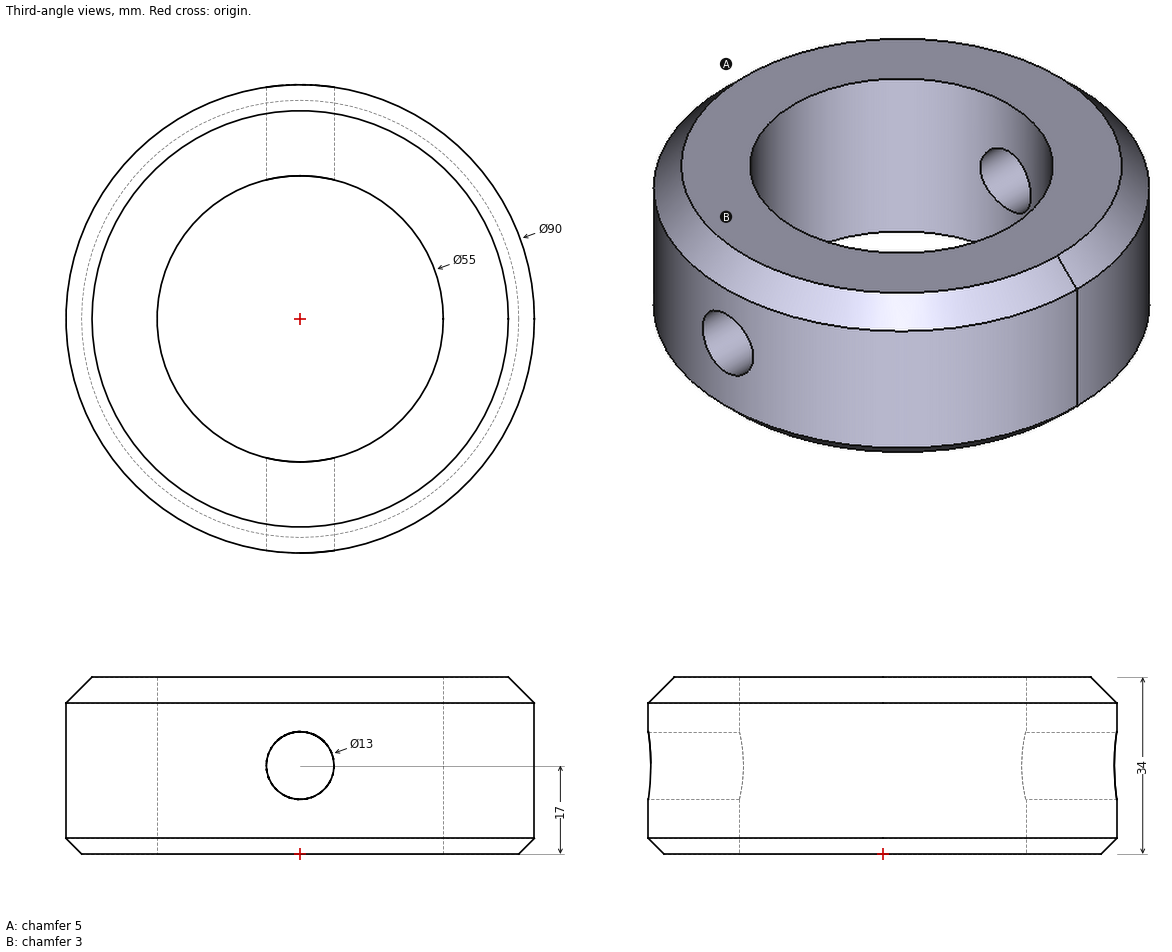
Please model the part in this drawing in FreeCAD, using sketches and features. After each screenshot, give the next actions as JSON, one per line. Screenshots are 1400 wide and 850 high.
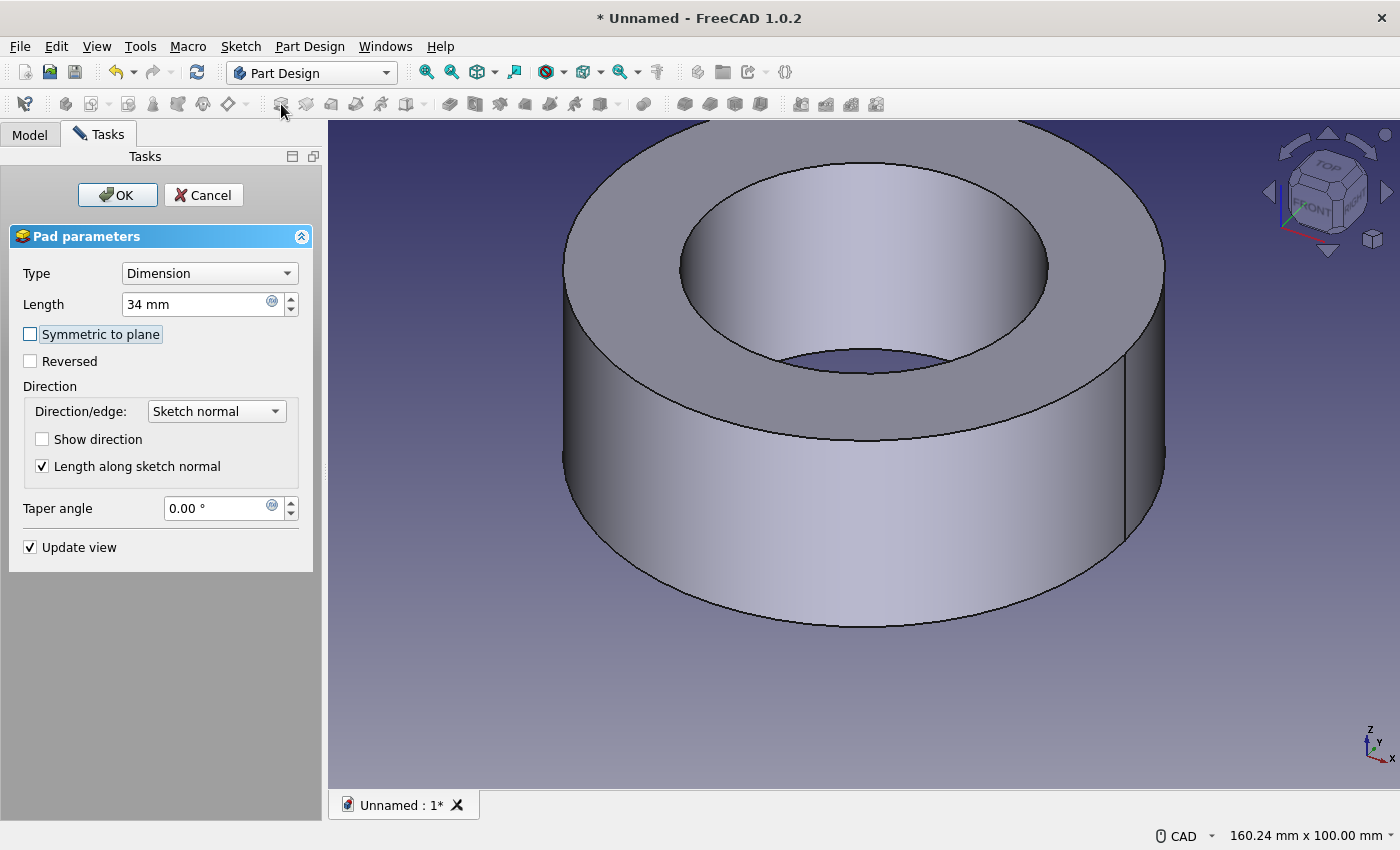
{"action": "left_click", "coordinate": [118, 195]}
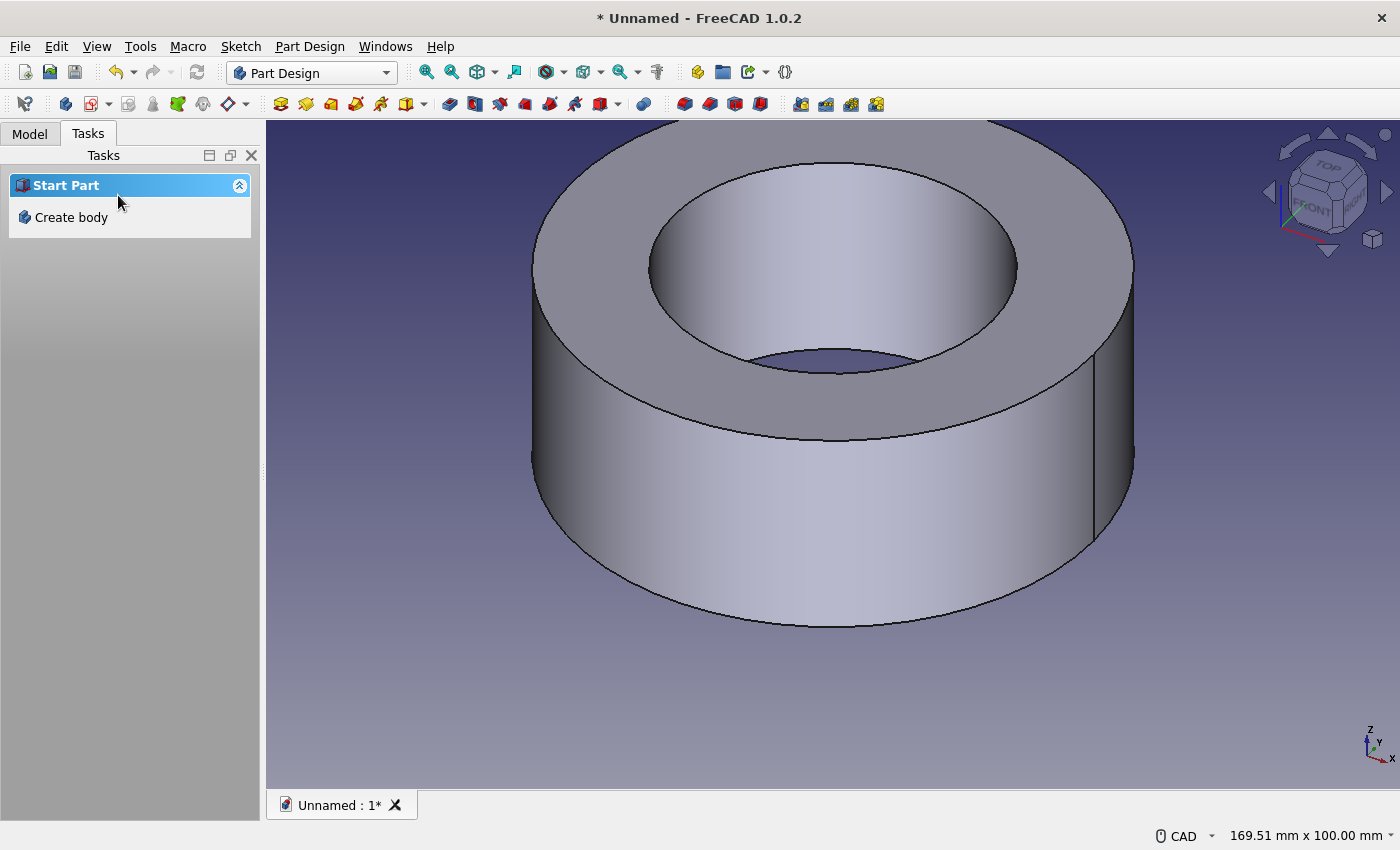
{"action": "left_click", "coordinate": [427, 72]}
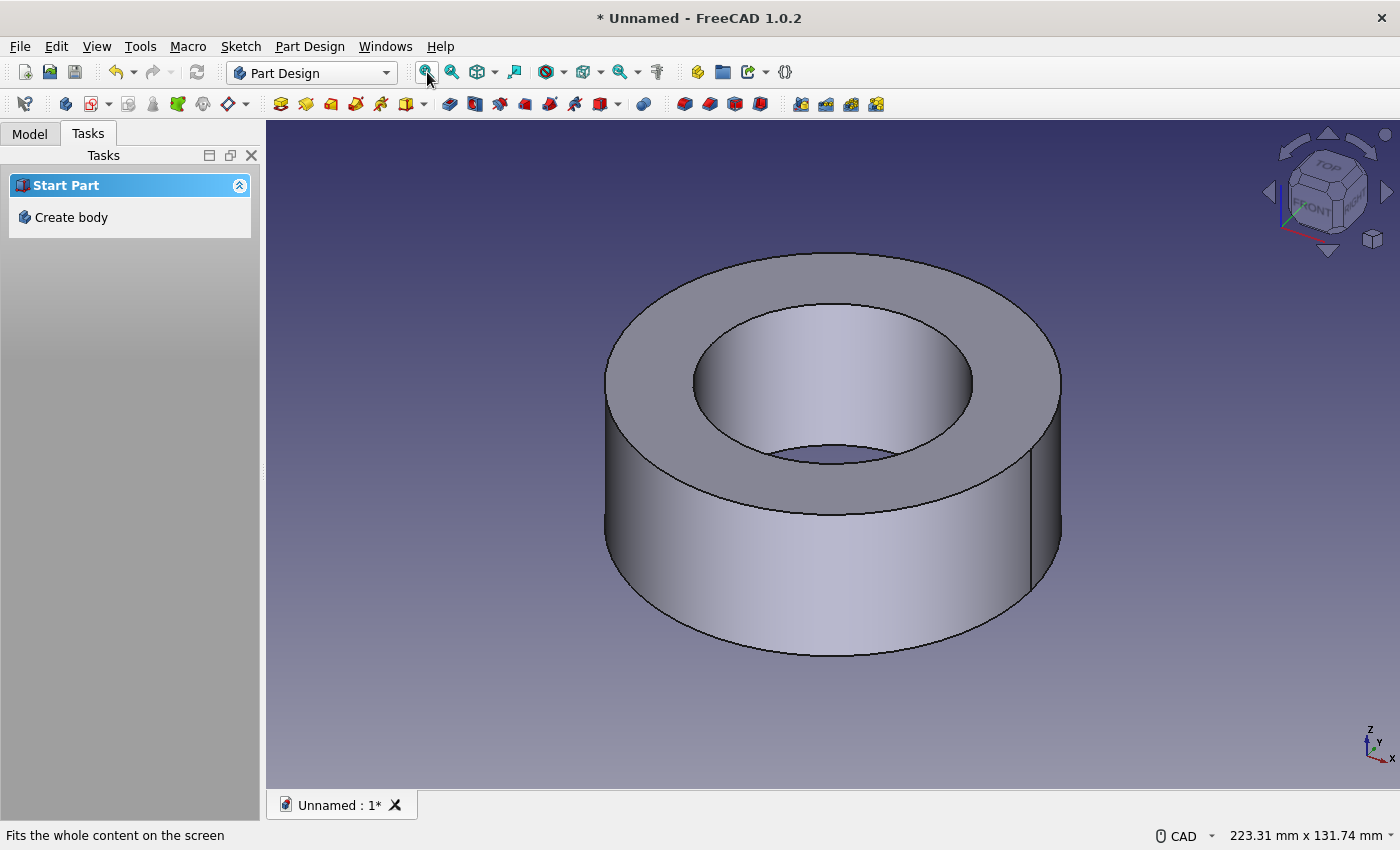
{"action": "left_click", "coordinate": [90, 104]}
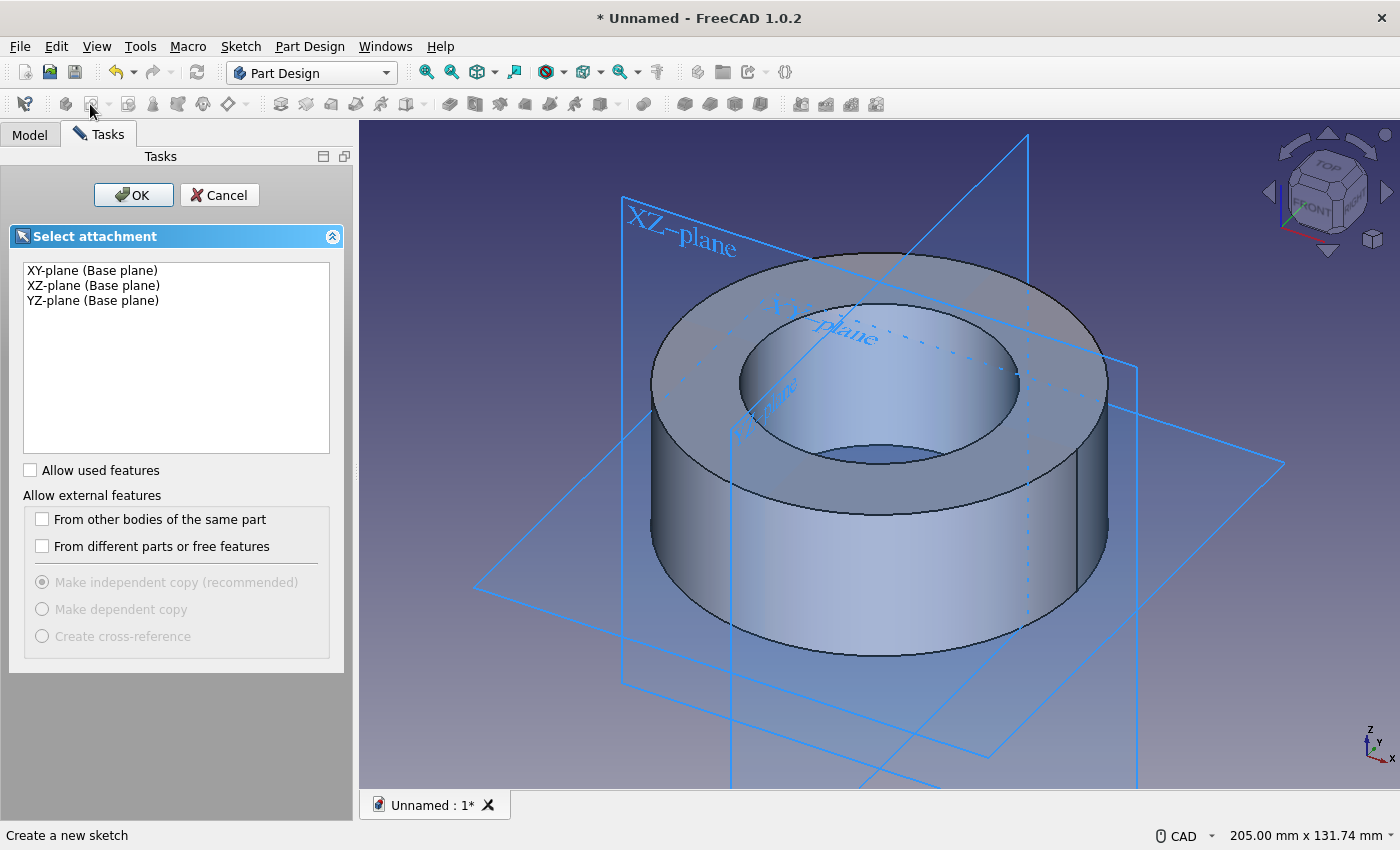
{"action": "left_click", "coordinate": [84, 286]}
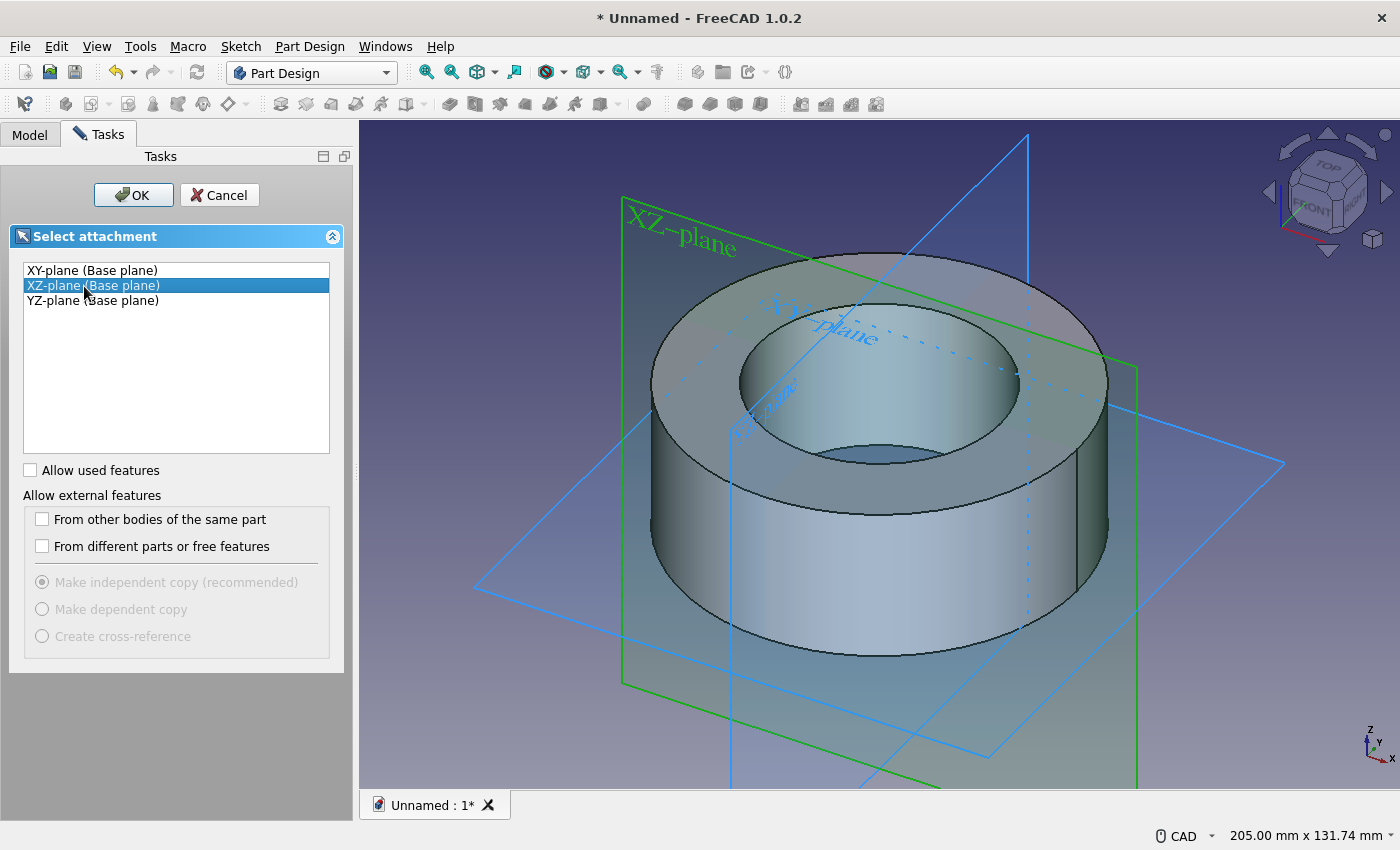
{"action": "left_click", "coordinate": [134, 195]}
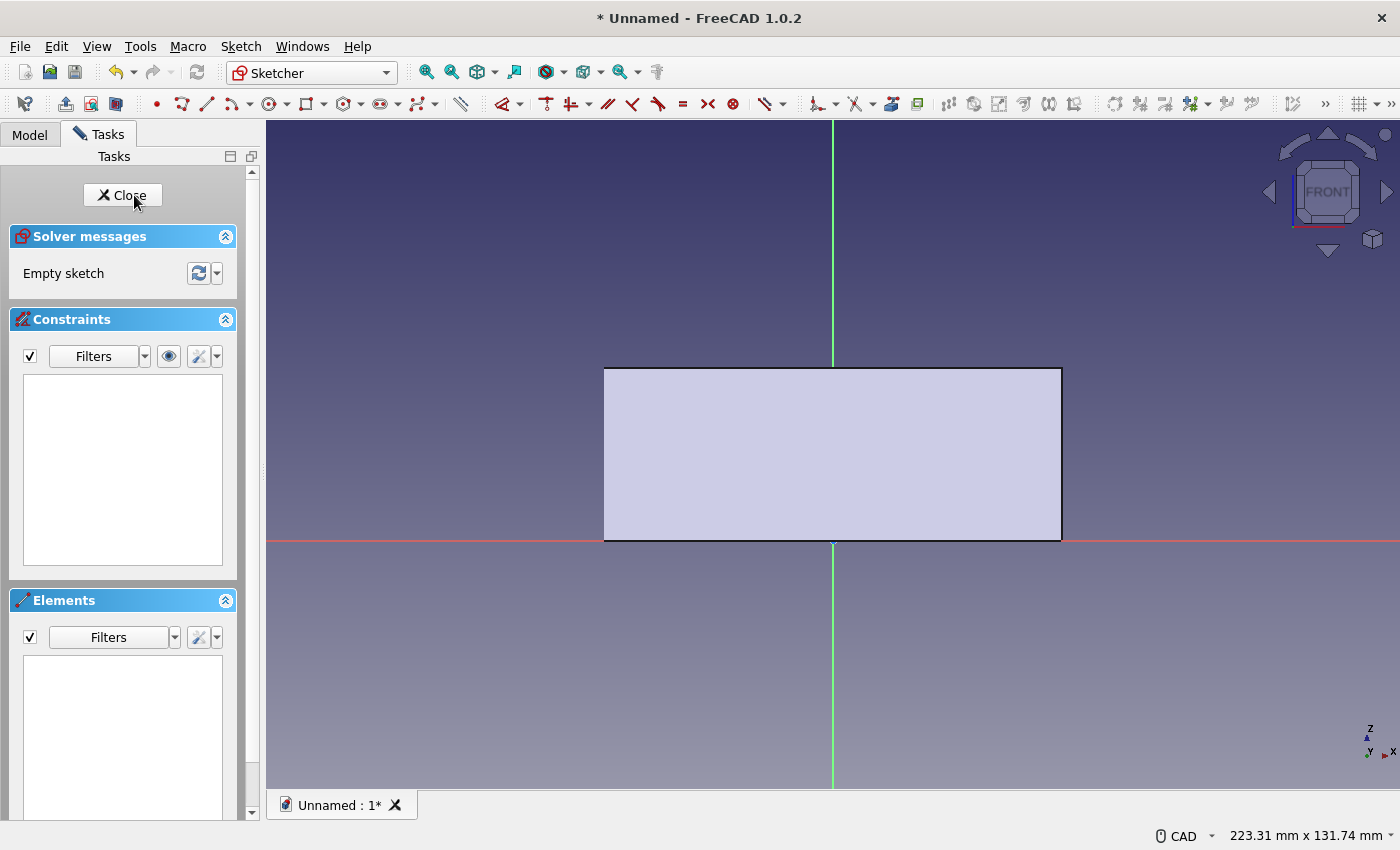
{"action": "key", "text": "q s"}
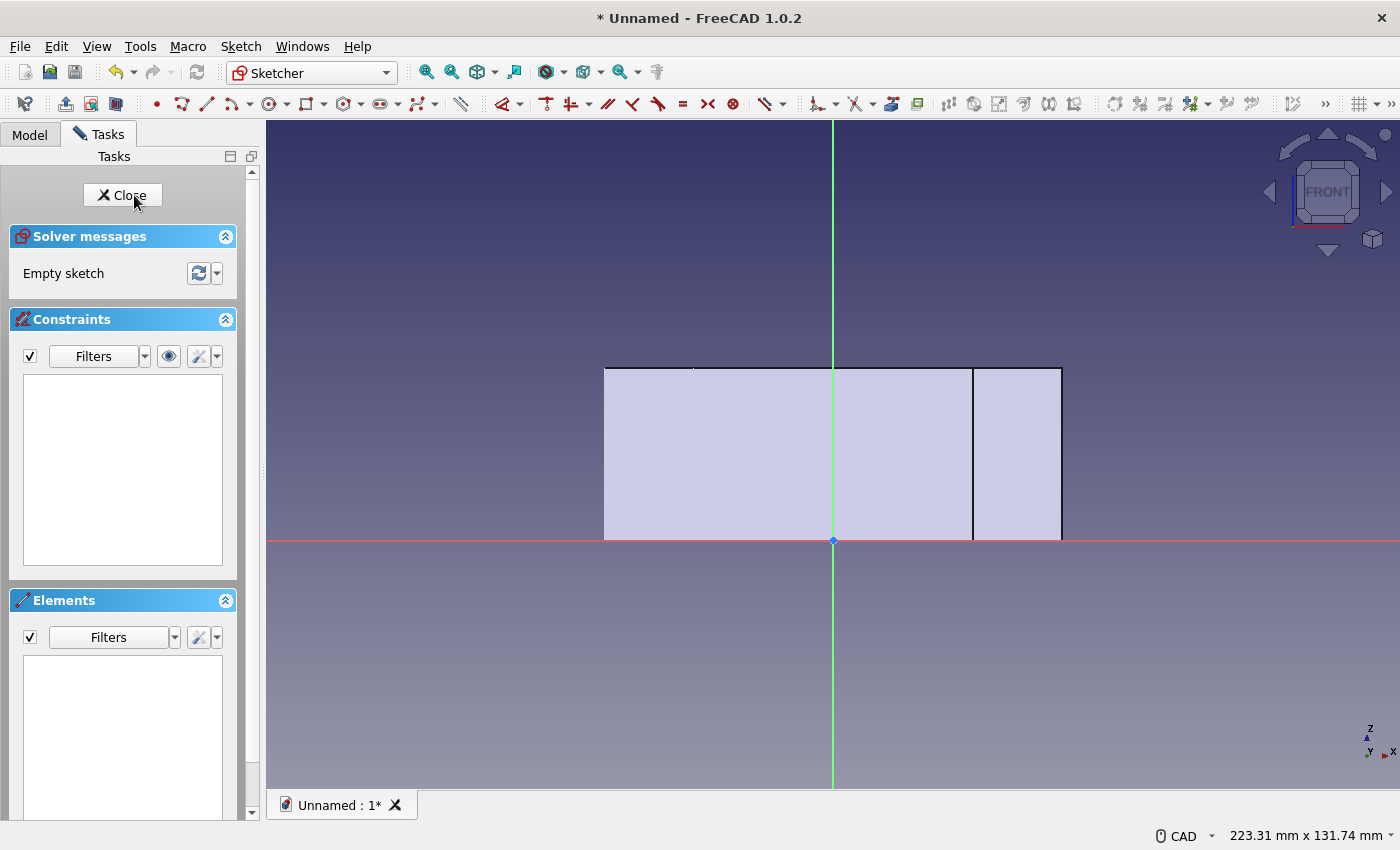
{"action": "scroll", "coordinate": [863, 493], "scroll_direction": "up", "scroll_amount": 6}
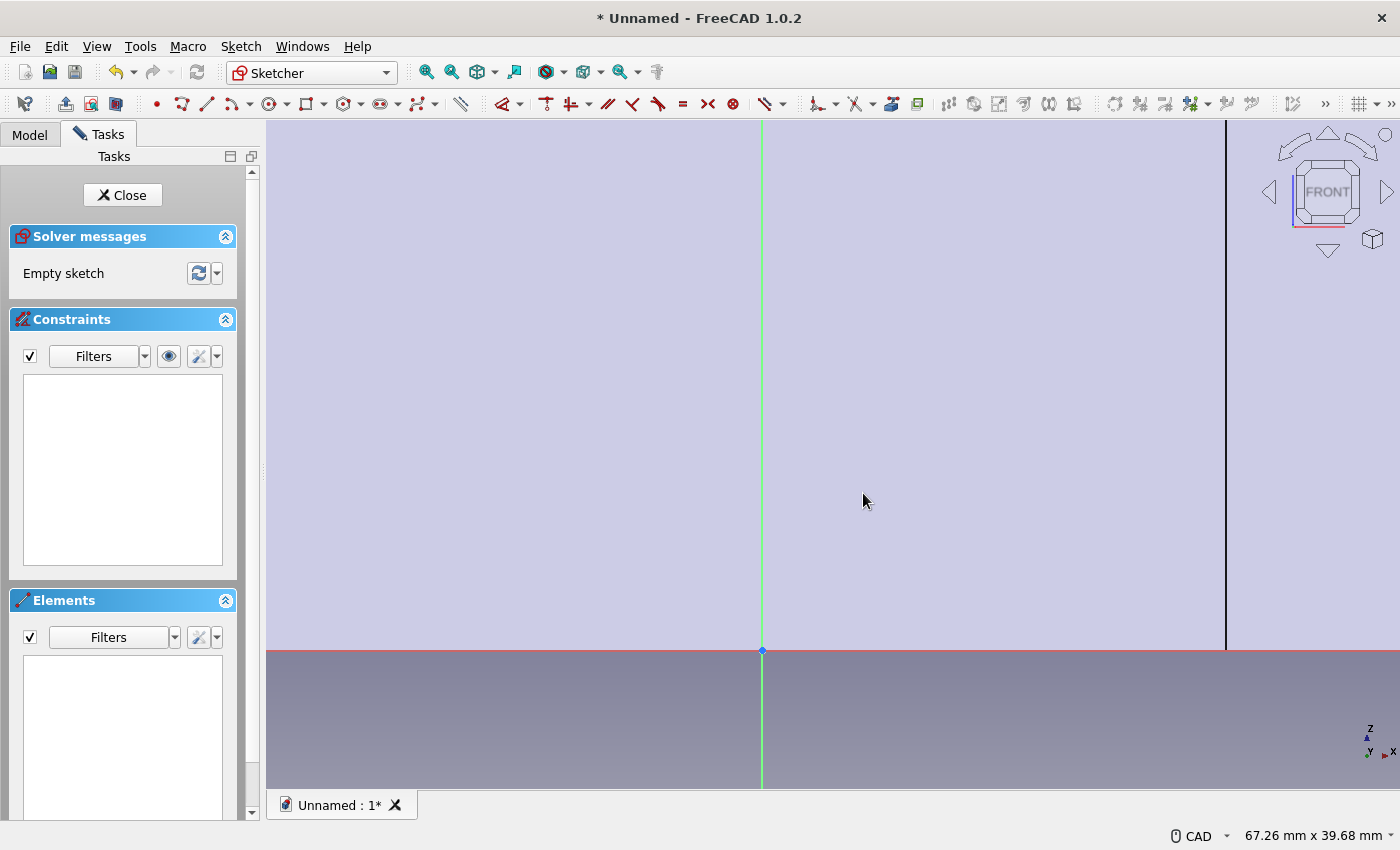
{"action": "key", "text": "g c"}